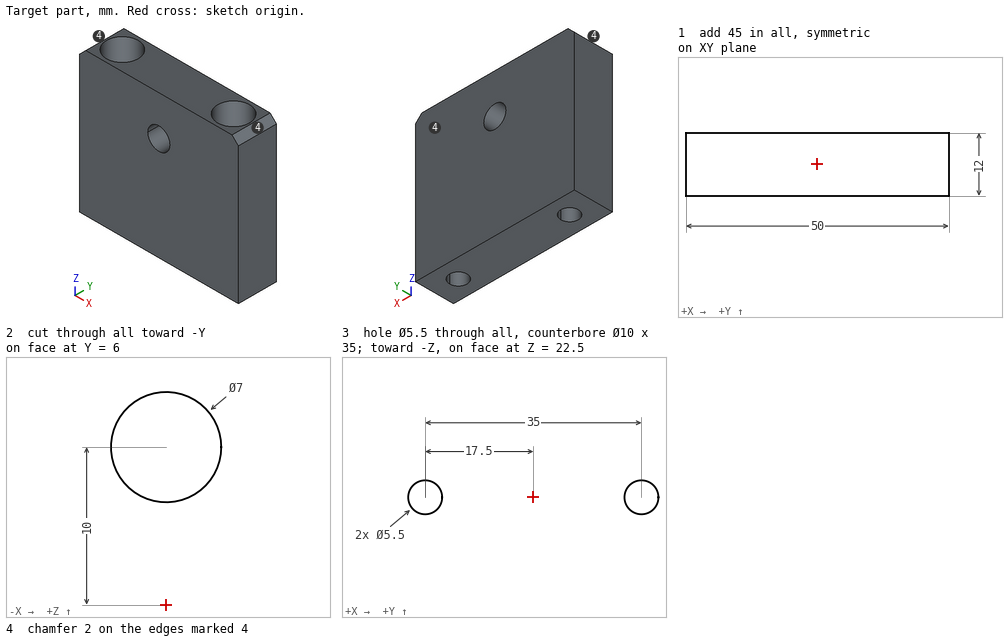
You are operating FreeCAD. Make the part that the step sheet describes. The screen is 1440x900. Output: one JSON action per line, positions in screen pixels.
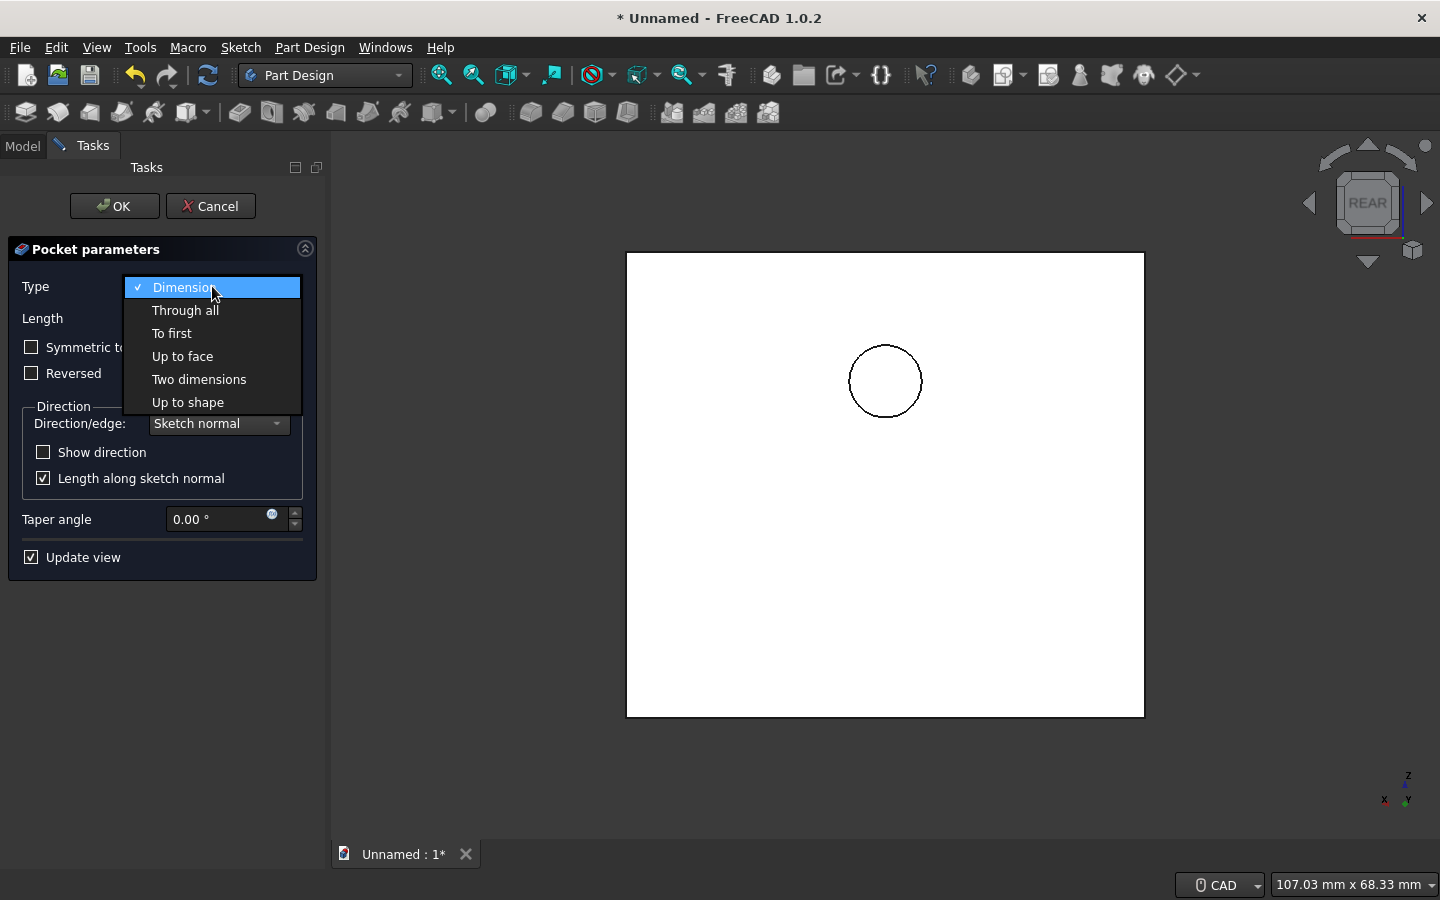
{"action": "left_click", "coordinate": [212, 310]}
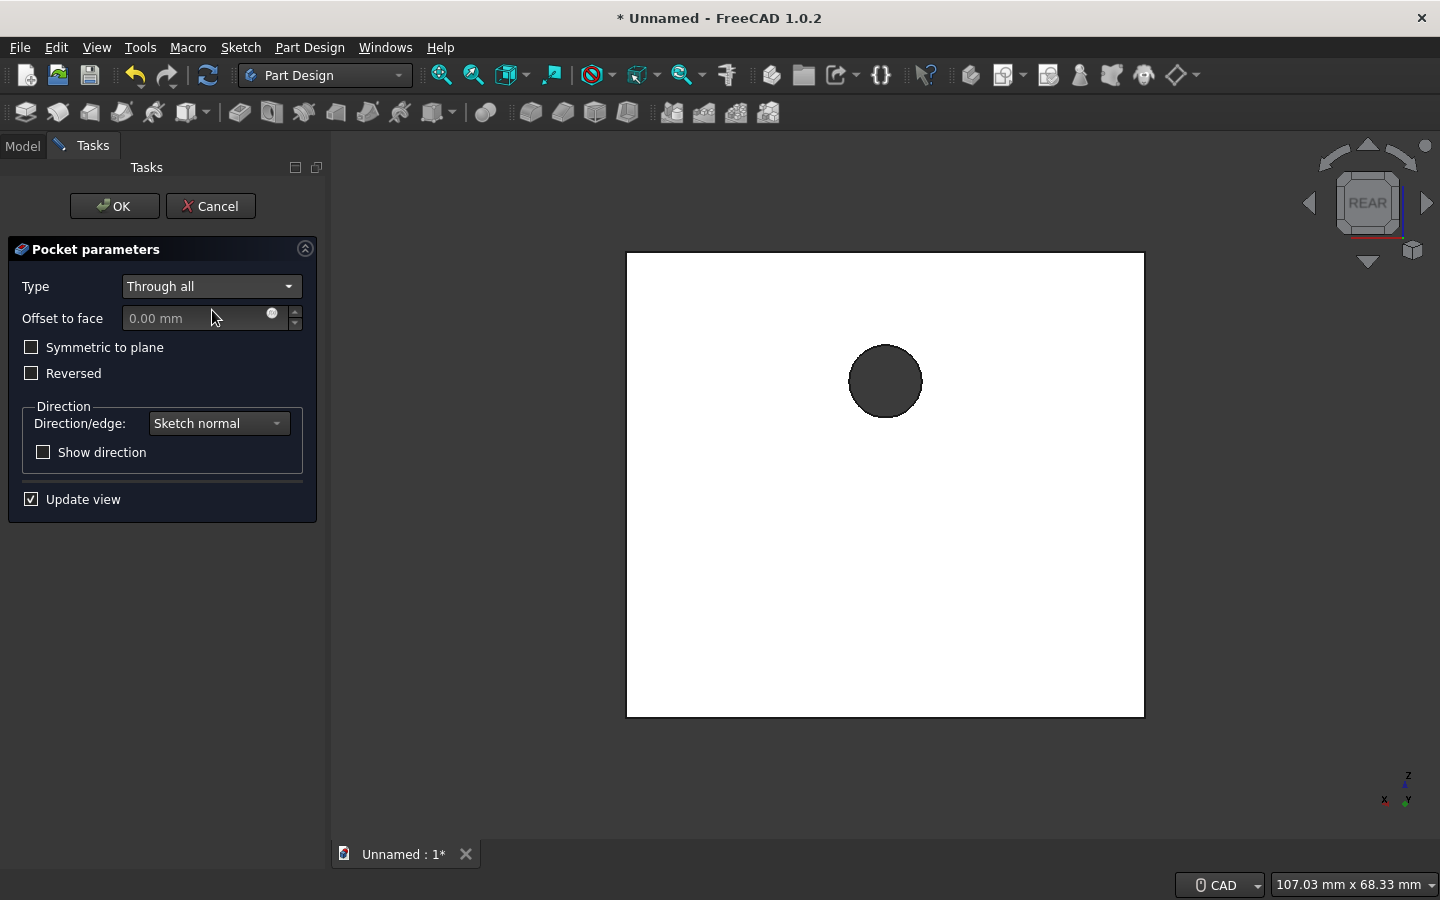
{"action": "left_click", "coordinate": [115, 206]}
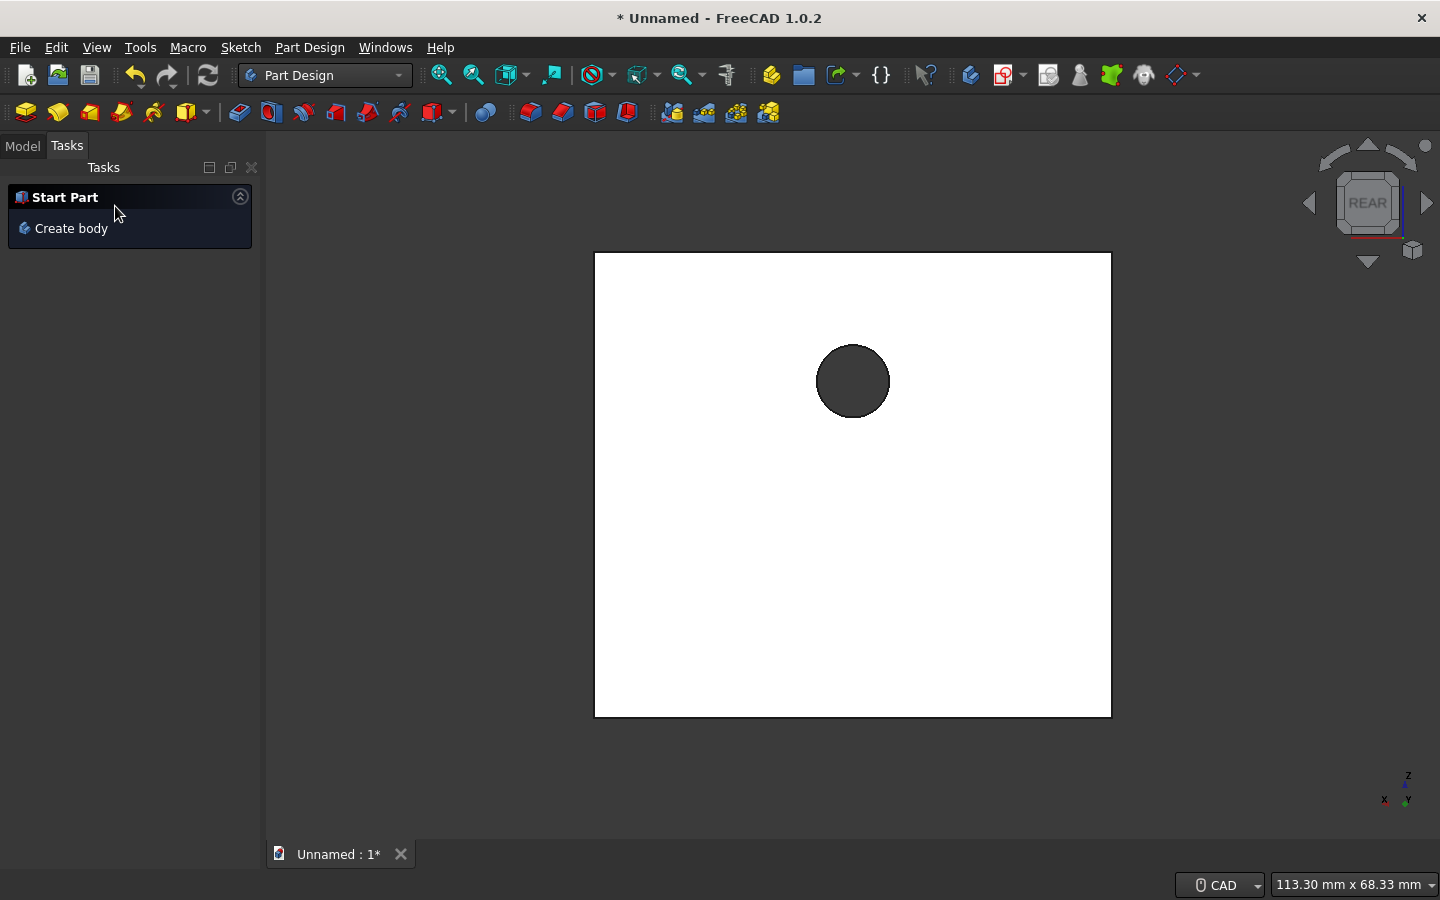
{"action": "key", "text": "0"}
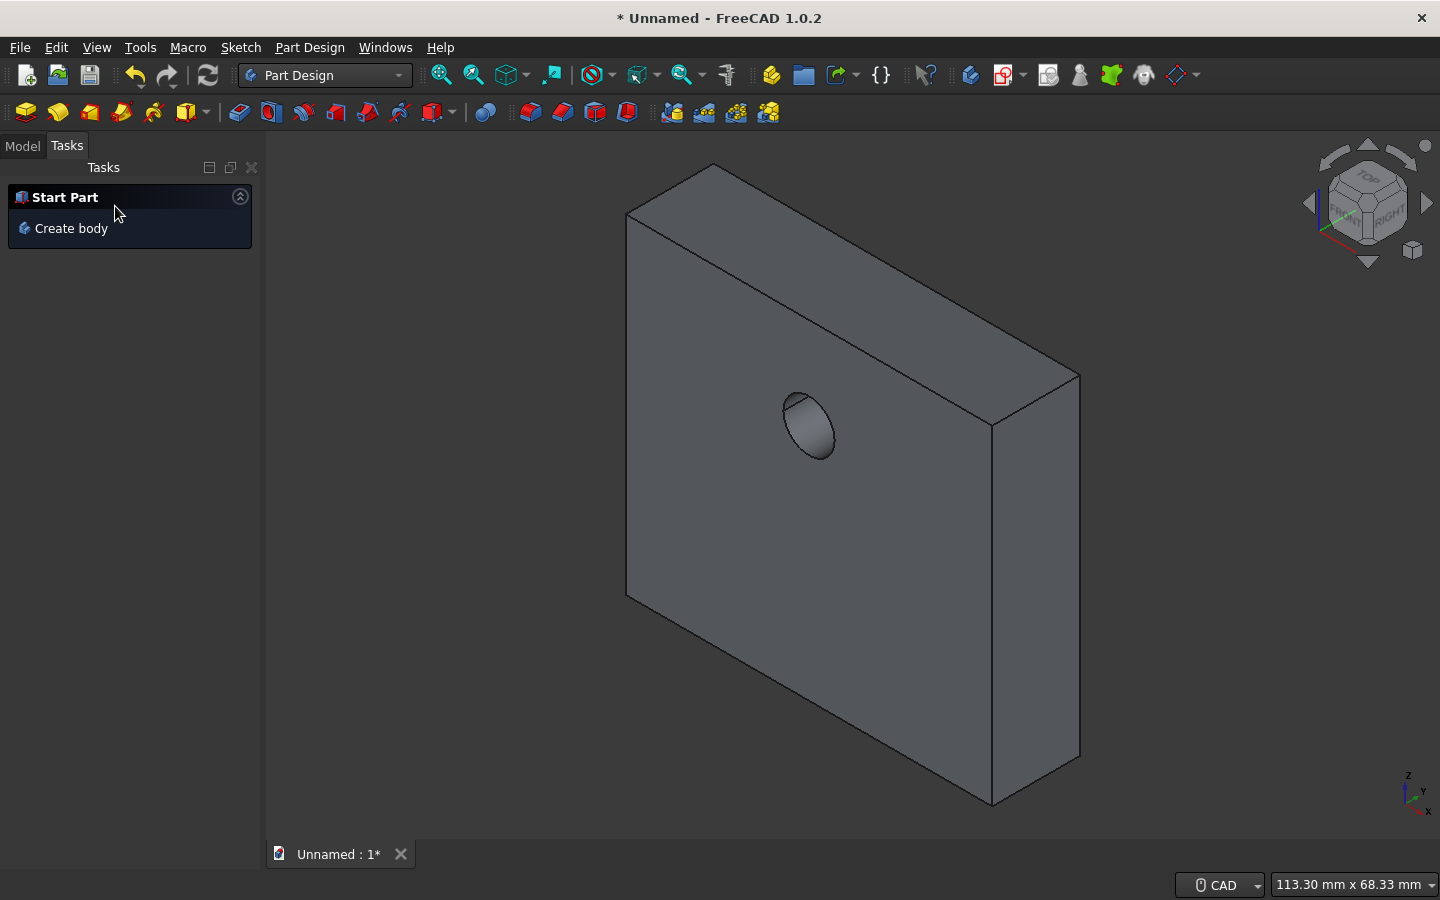
{"action": "left_click", "coordinate": [958, 354]}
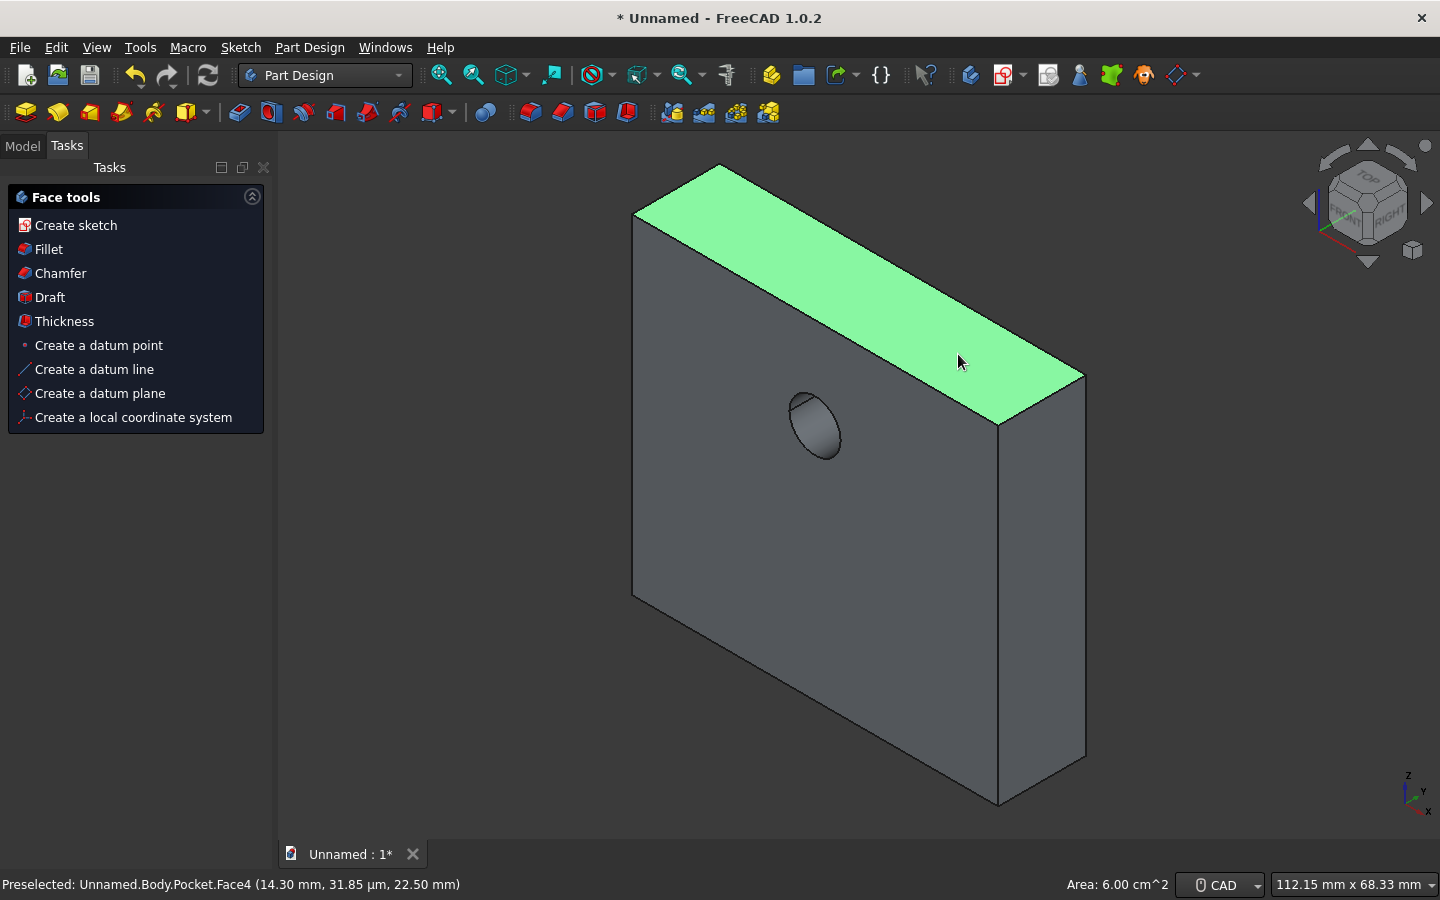
{"action": "left_click", "coordinate": [1004, 76]}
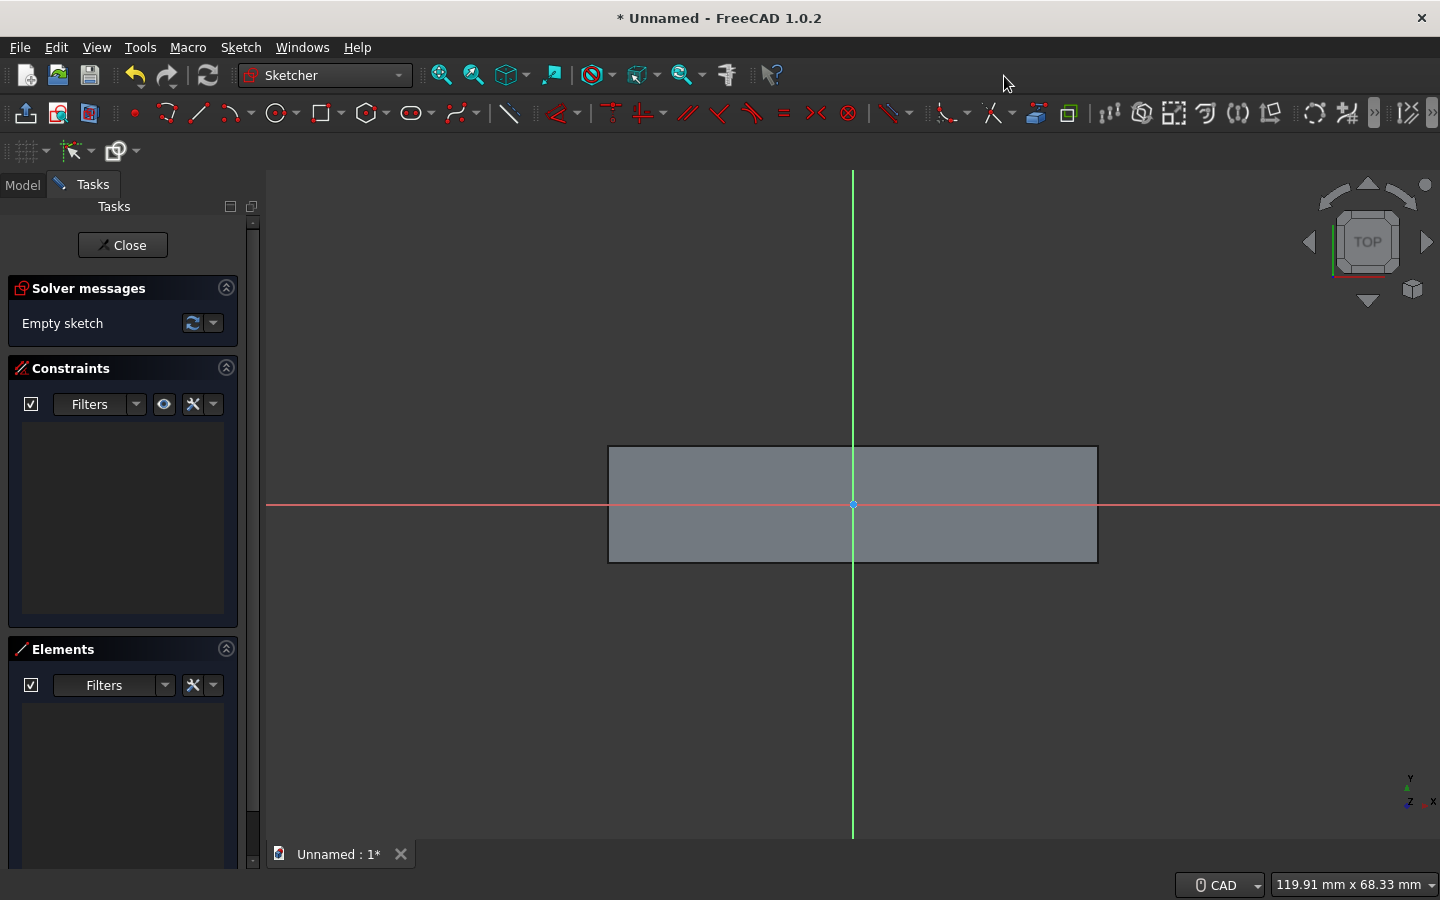
{"action": "scroll", "coordinate": [936, 504], "scroll_direction": "up", "scroll_amount": 3}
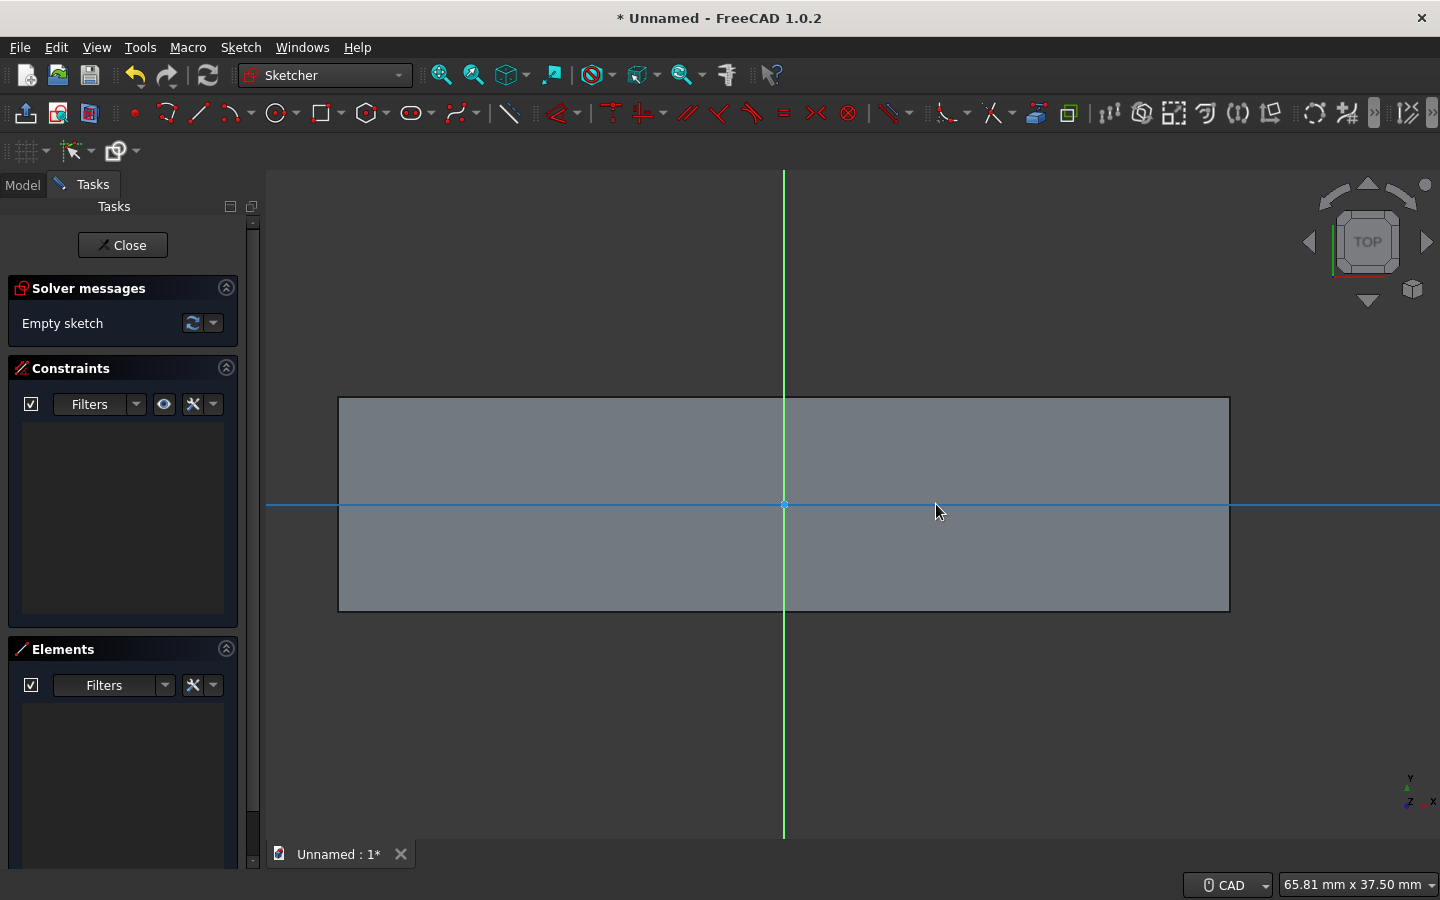
{"action": "left_click", "coordinate": [276, 114]}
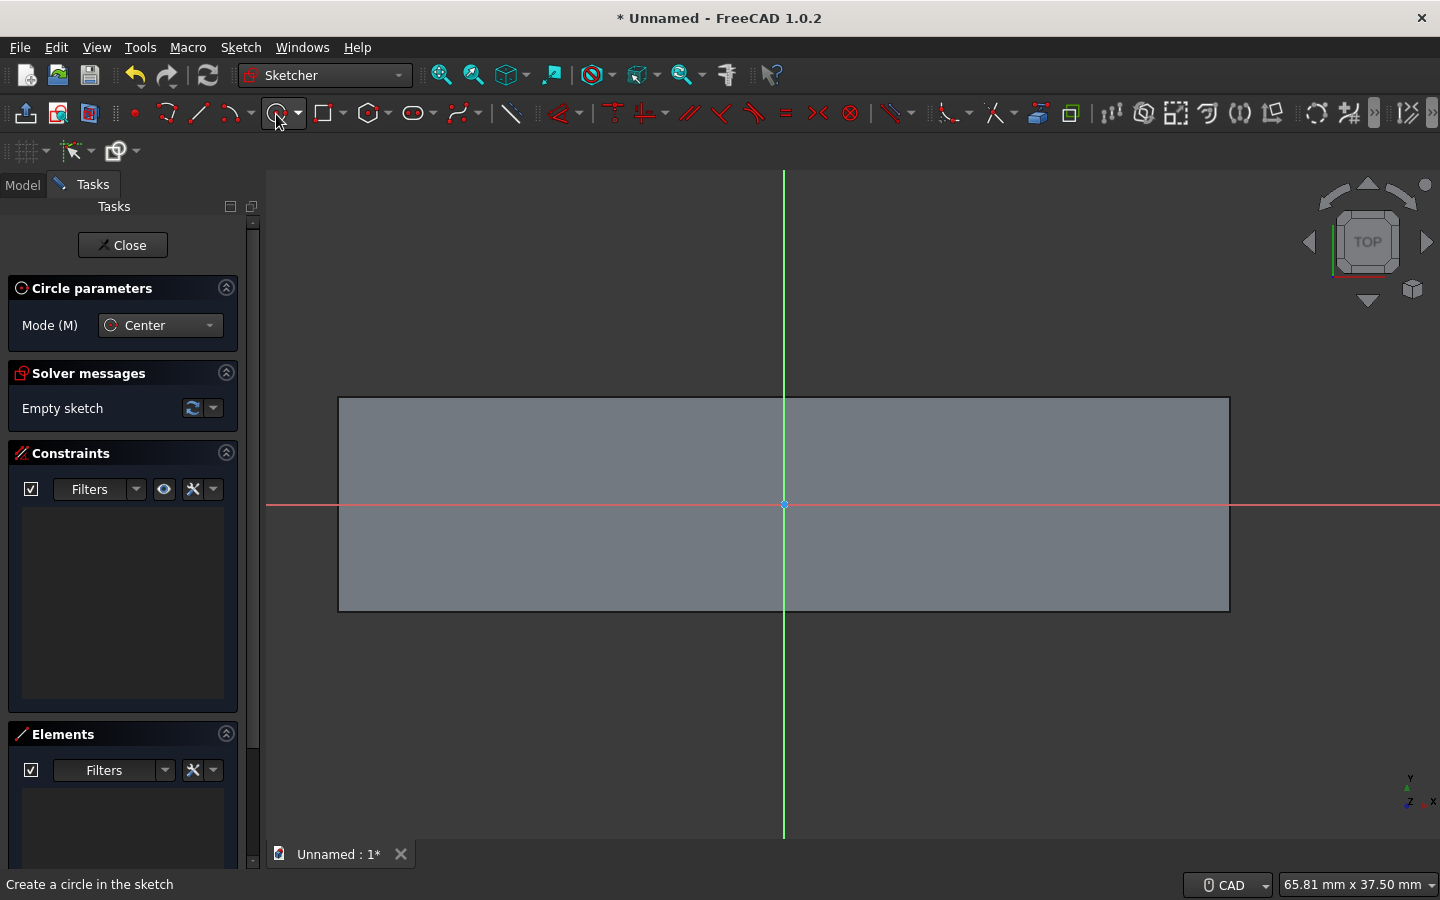
{"action": "left_click", "coordinate": [472, 504]}
{"action": "left_click", "coordinate": [507, 470]}